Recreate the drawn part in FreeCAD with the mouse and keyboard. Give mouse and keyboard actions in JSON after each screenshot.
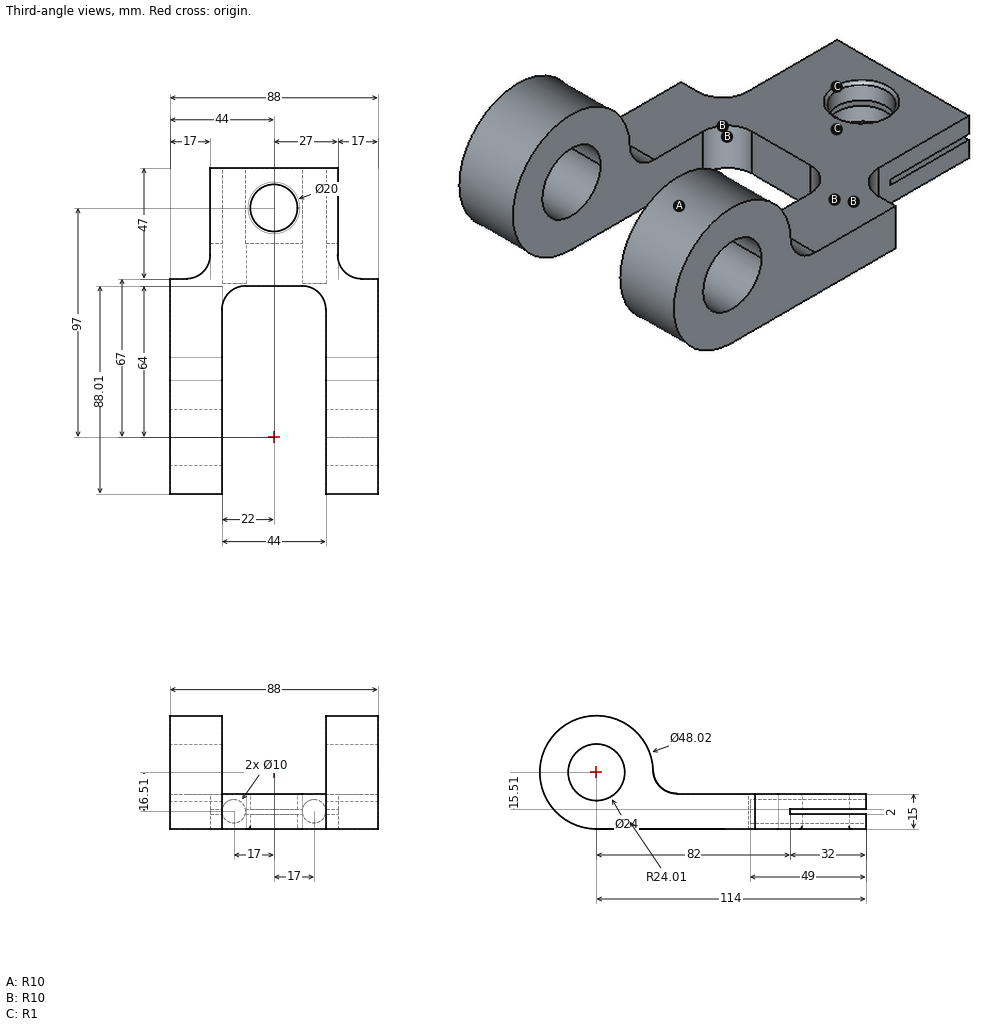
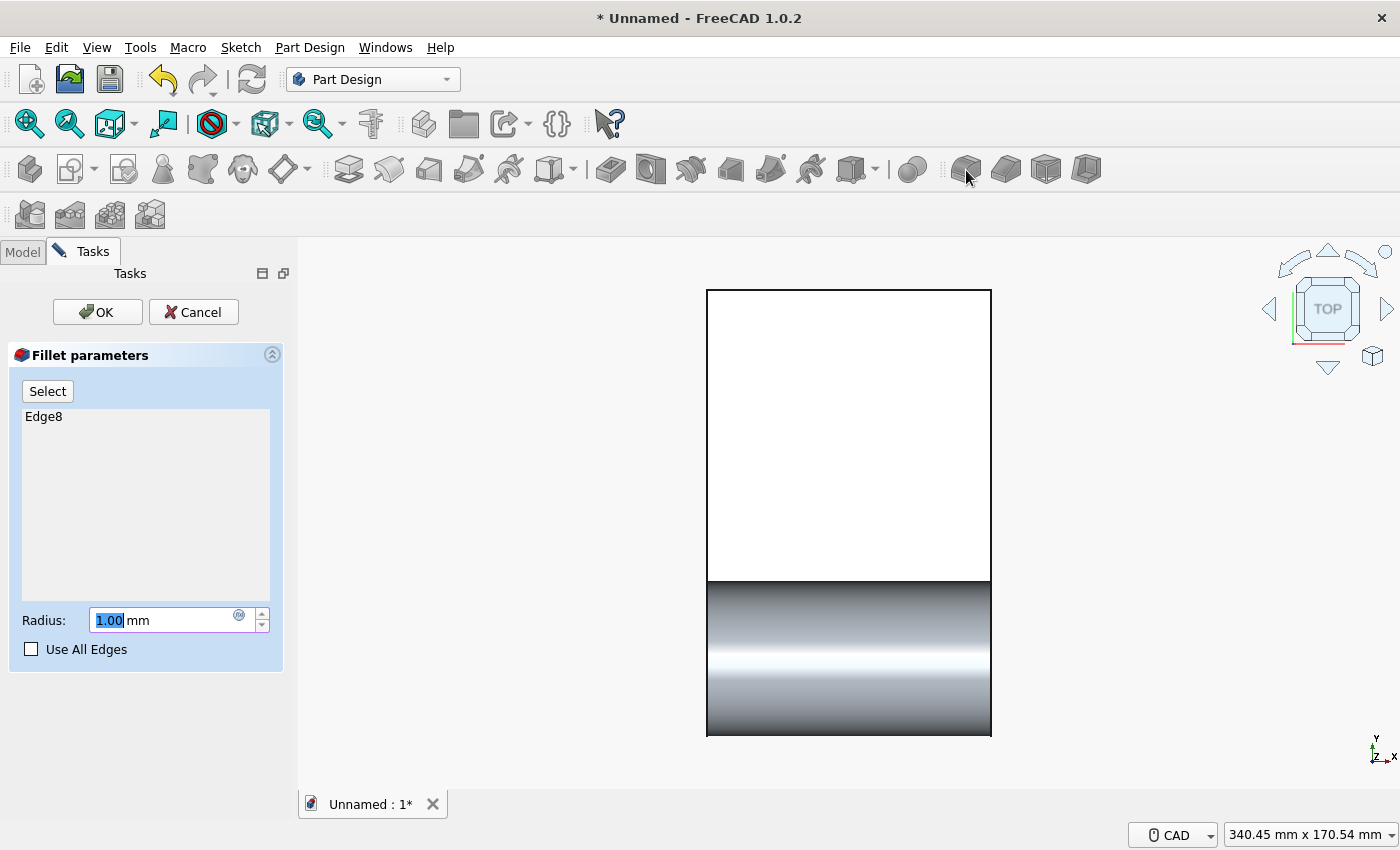
{"action": "type", "text": "10"}
{"action": "key", "text": "Tab"}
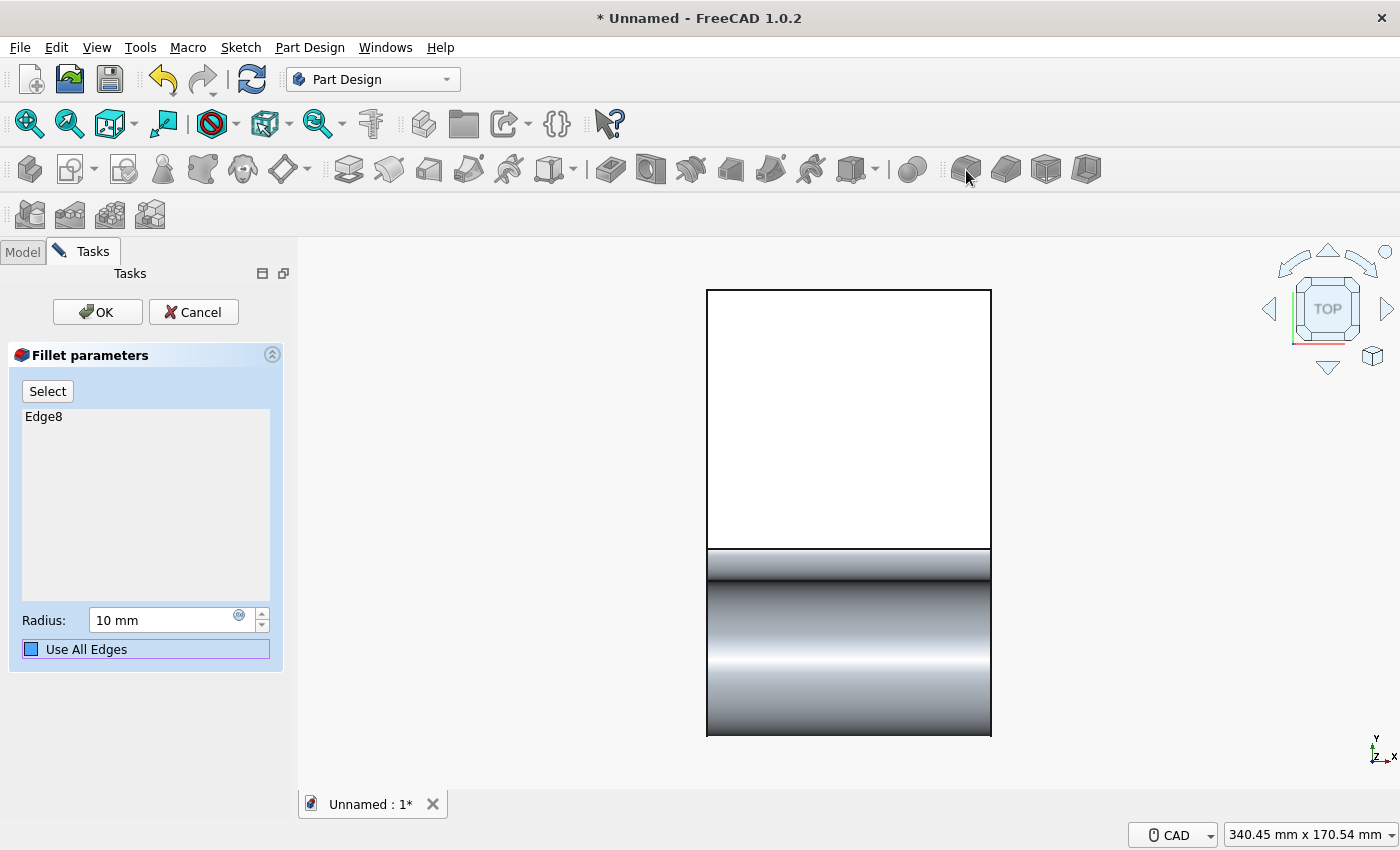
{"action": "left_click", "coordinate": [98, 312]}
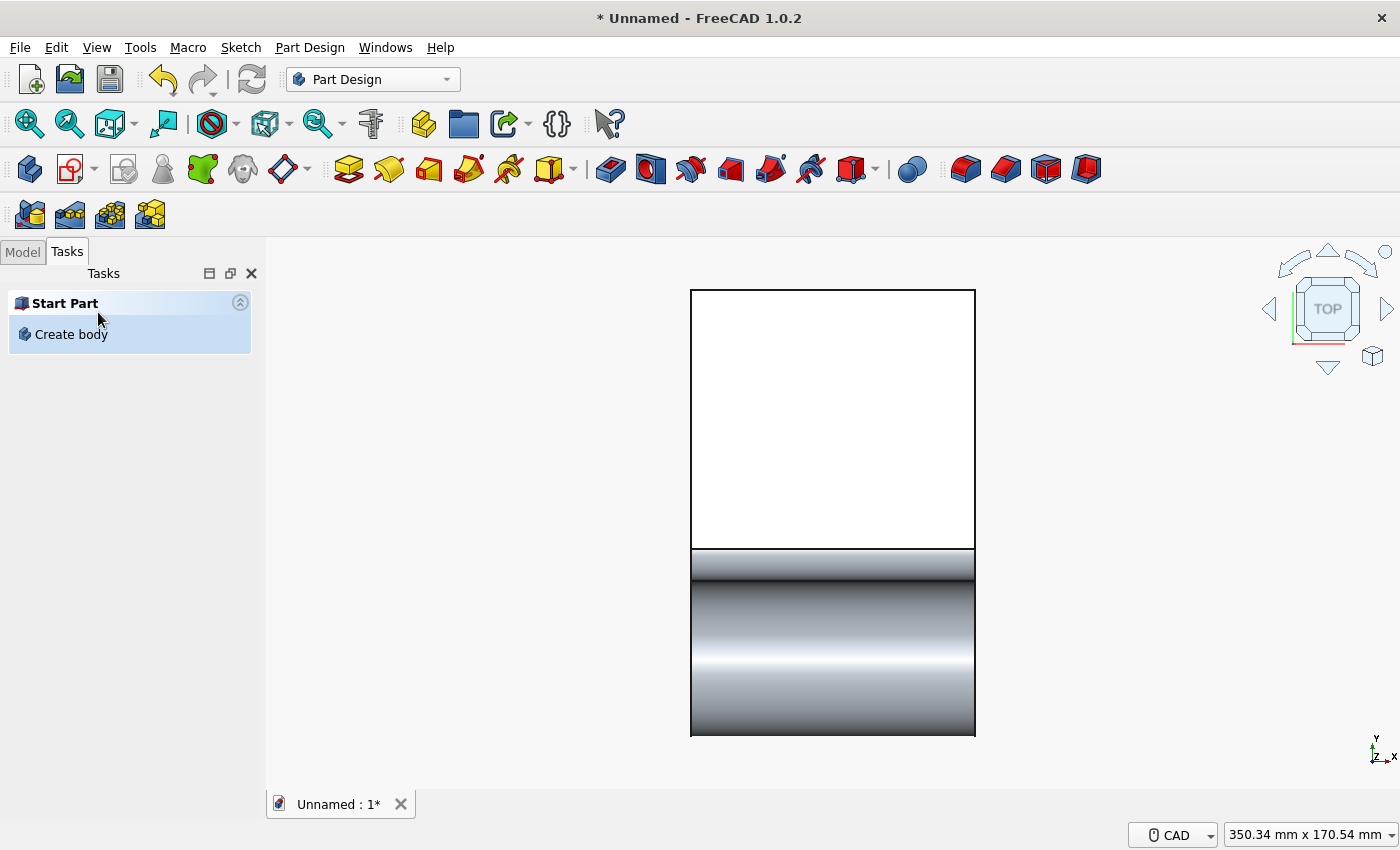
{"action": "left_click", "coordinate": [70, 170]}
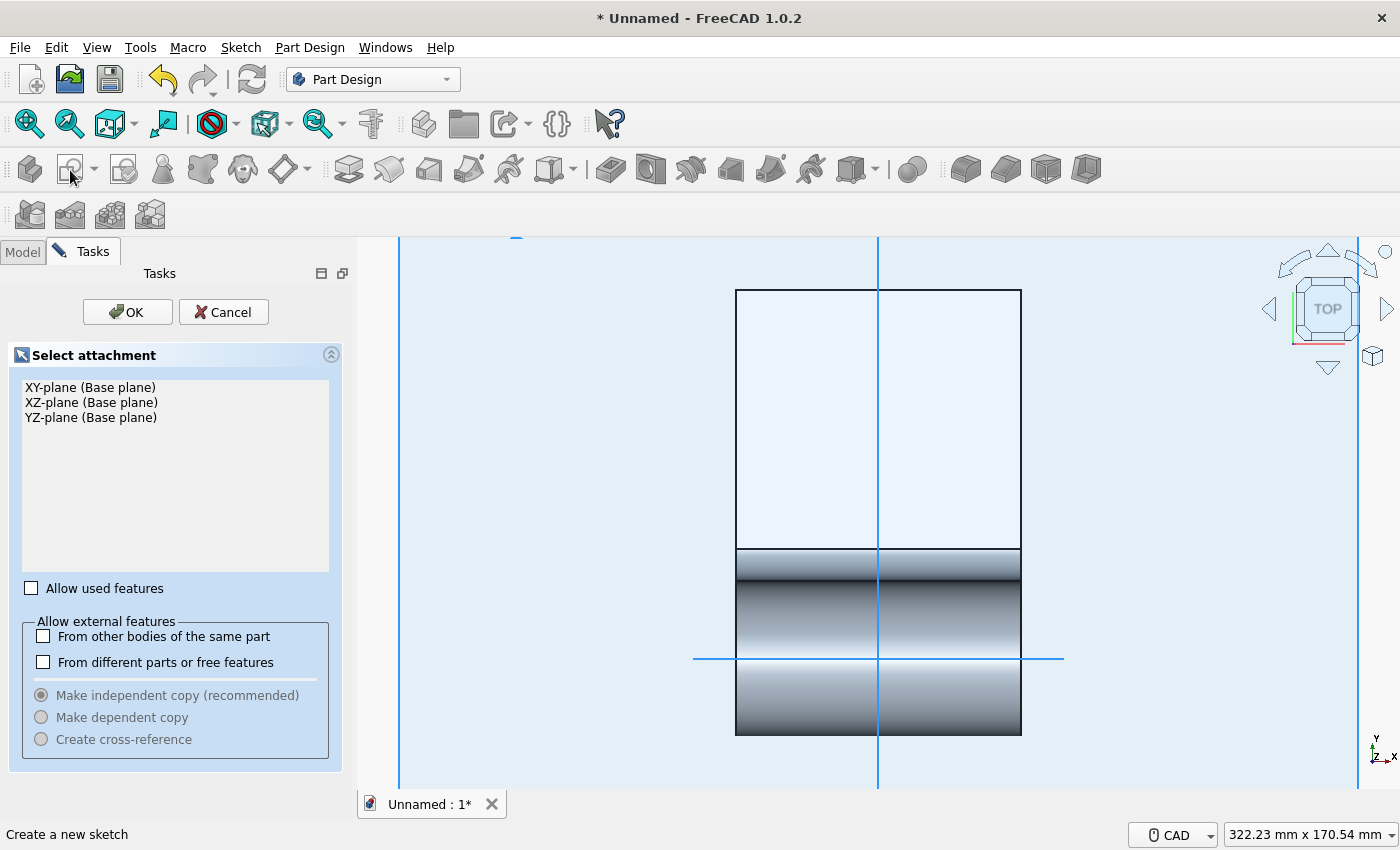
{"action": "left_click", "coordinate": [82, 388]}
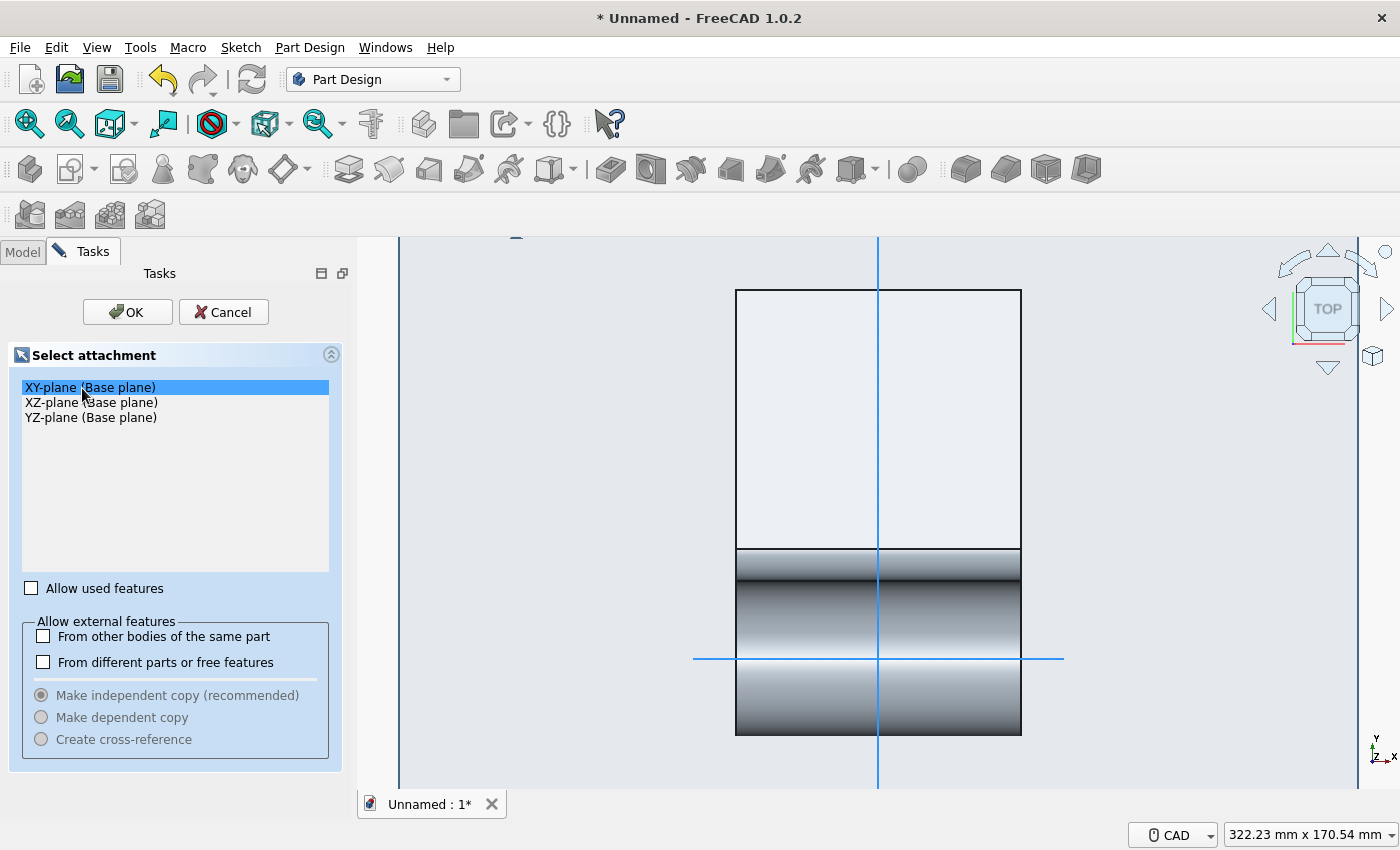
{"action": "left_click", "coordinate": [128, 312]}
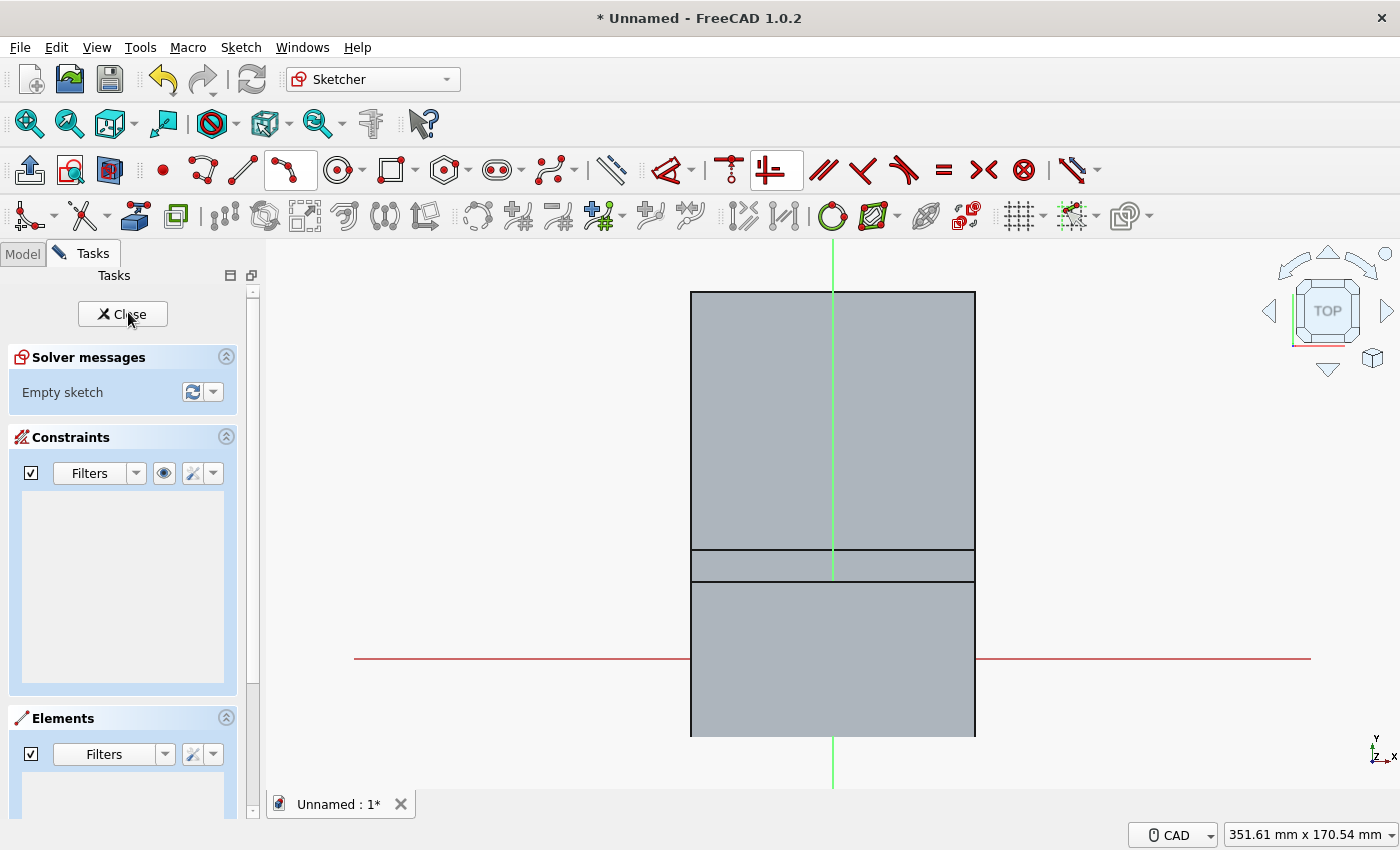
{"action": "left_click", "coordinate": [110, 170]}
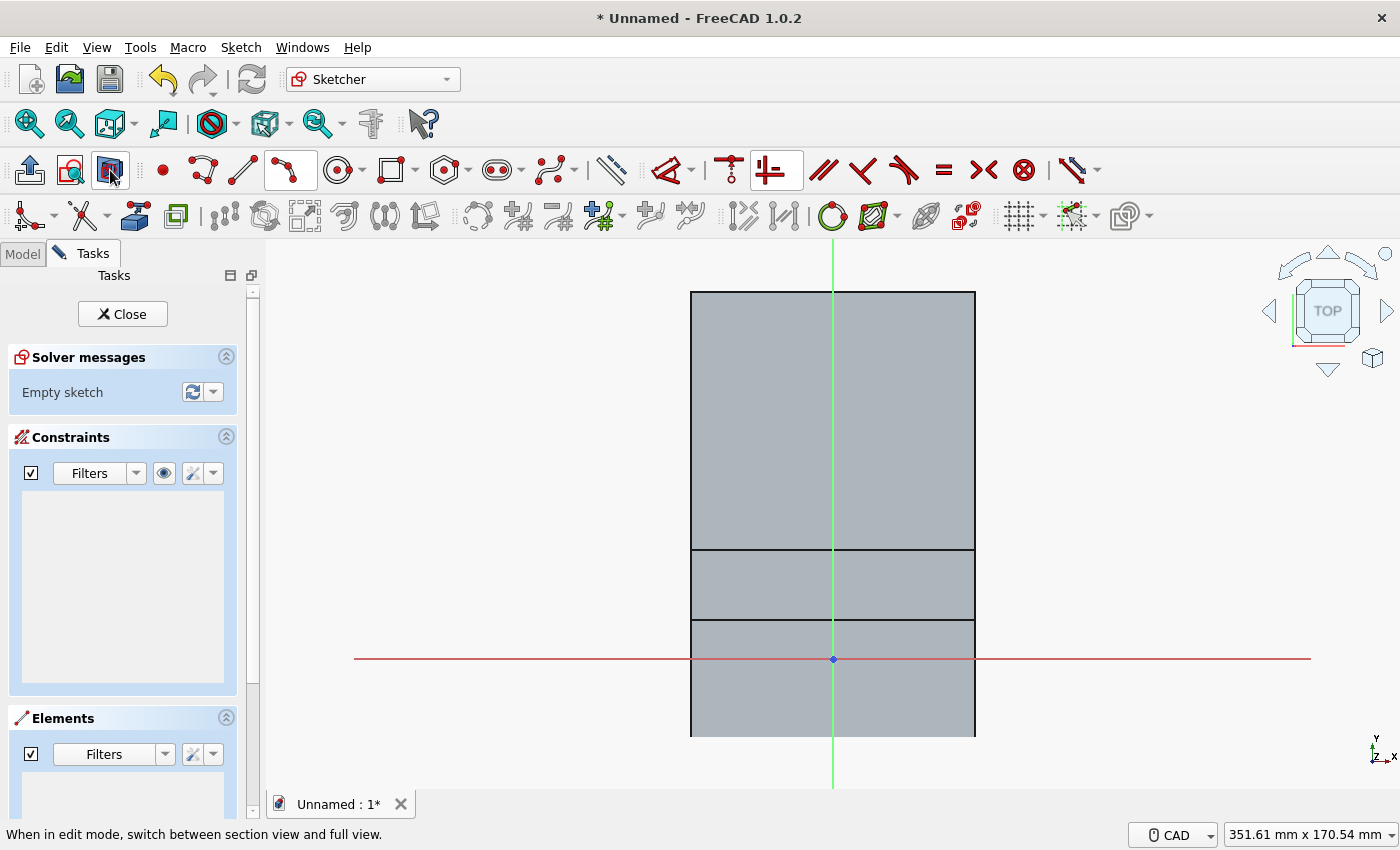
{"action": "scroll", "coordinate": [1142, 761], "scroll_direction": "up", "scroll_amount": 1}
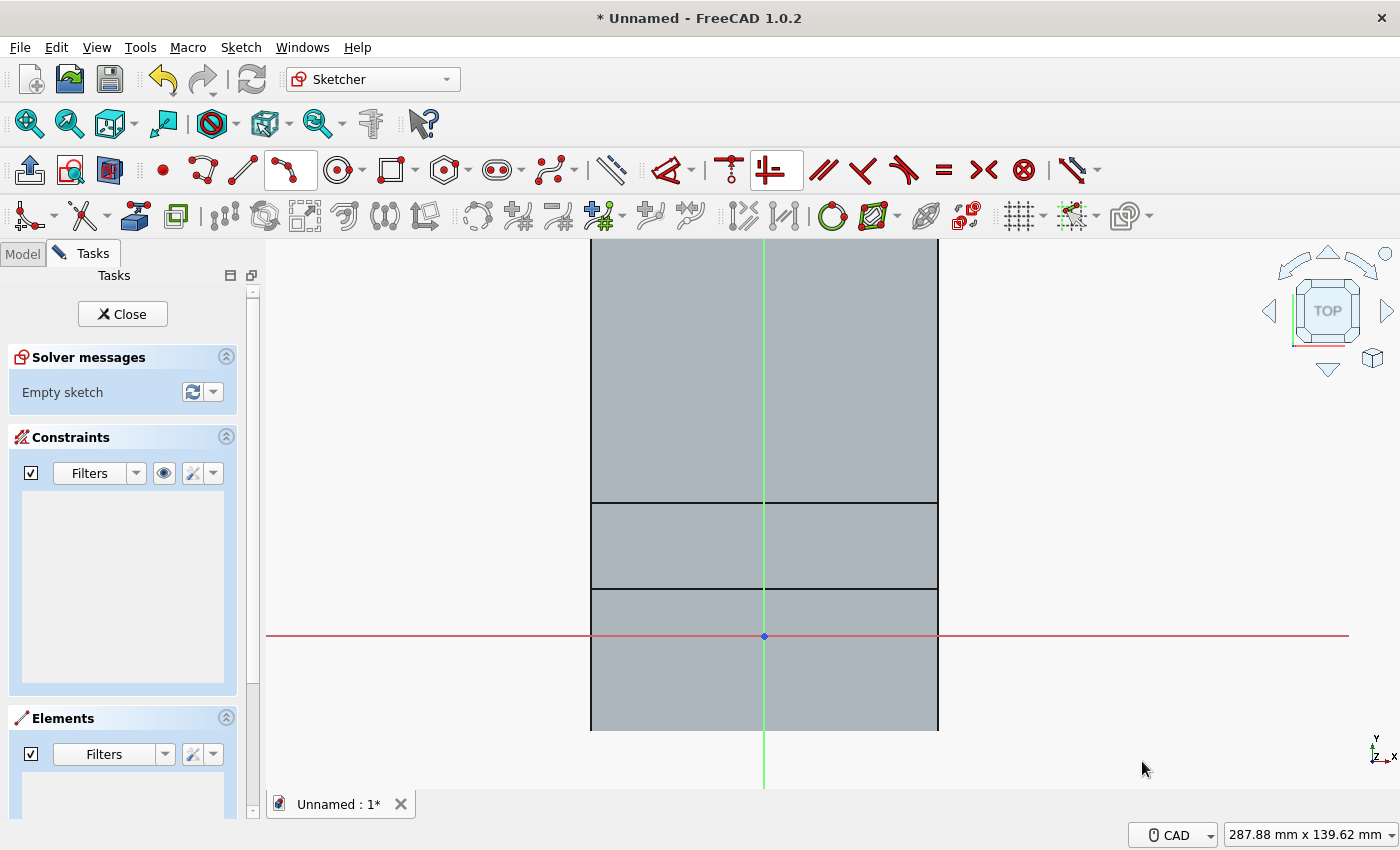
{"action": "left_click", "coordinate": [392, 170]}